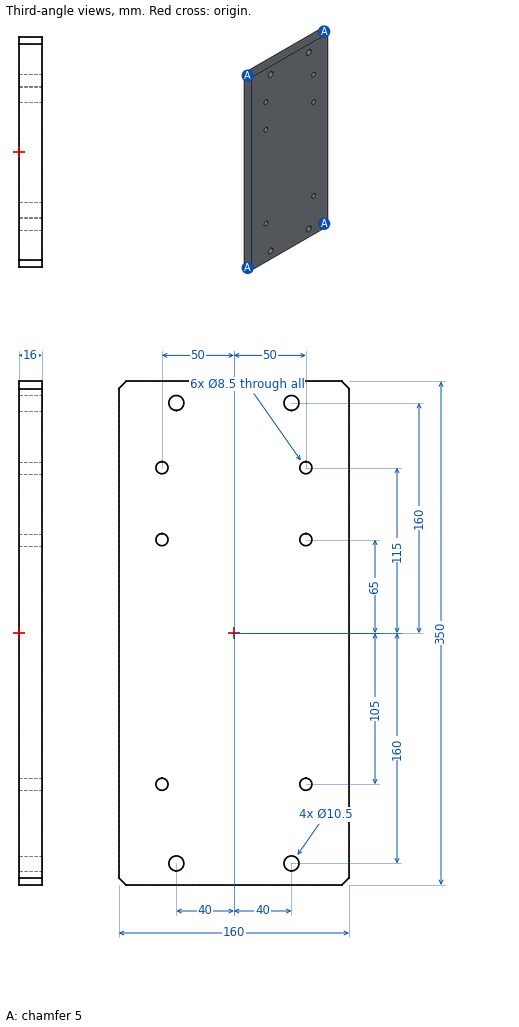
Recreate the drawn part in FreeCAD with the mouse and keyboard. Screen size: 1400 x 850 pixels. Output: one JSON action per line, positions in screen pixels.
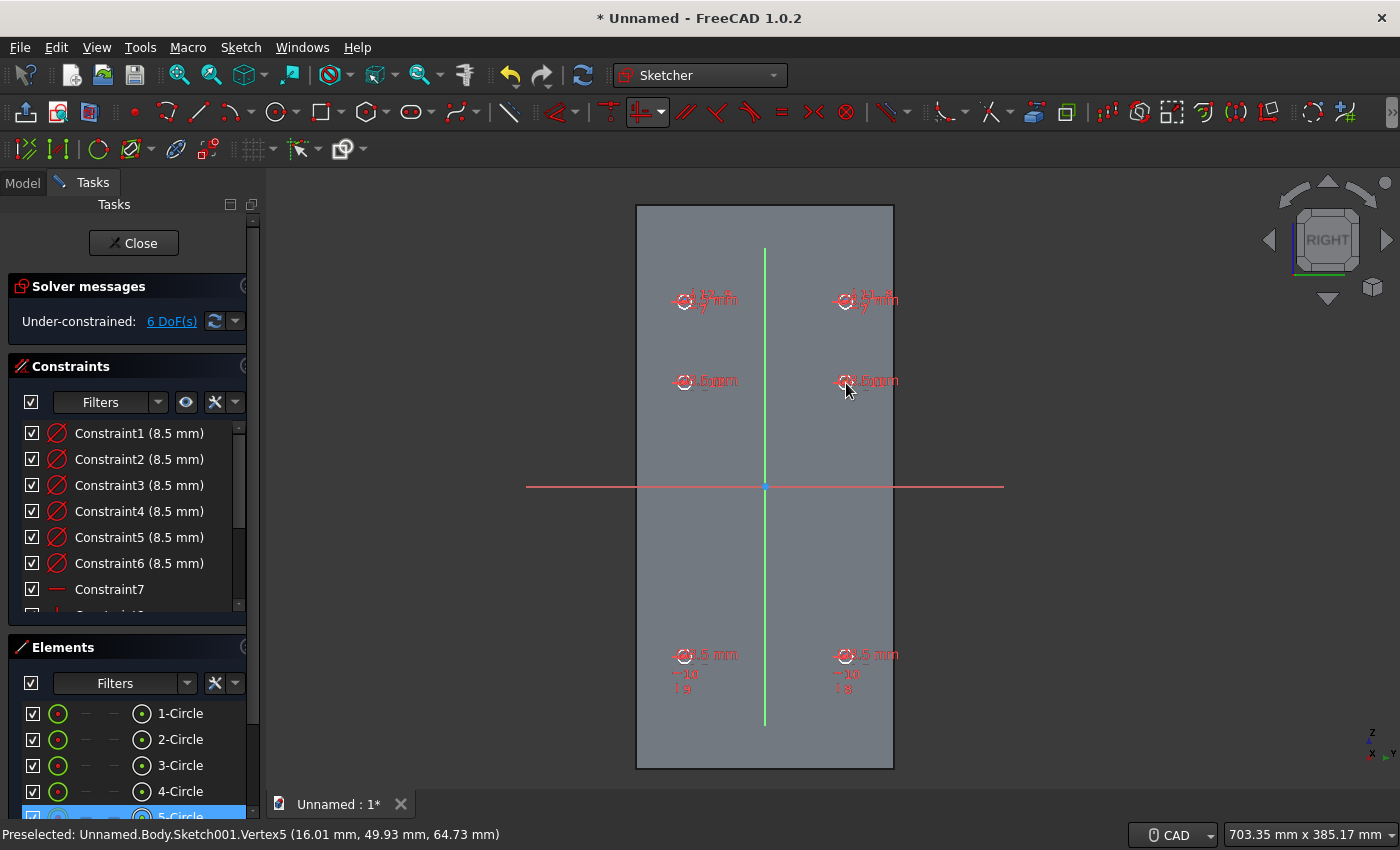
{"action": "left_click", "coordinate": [685, 383]}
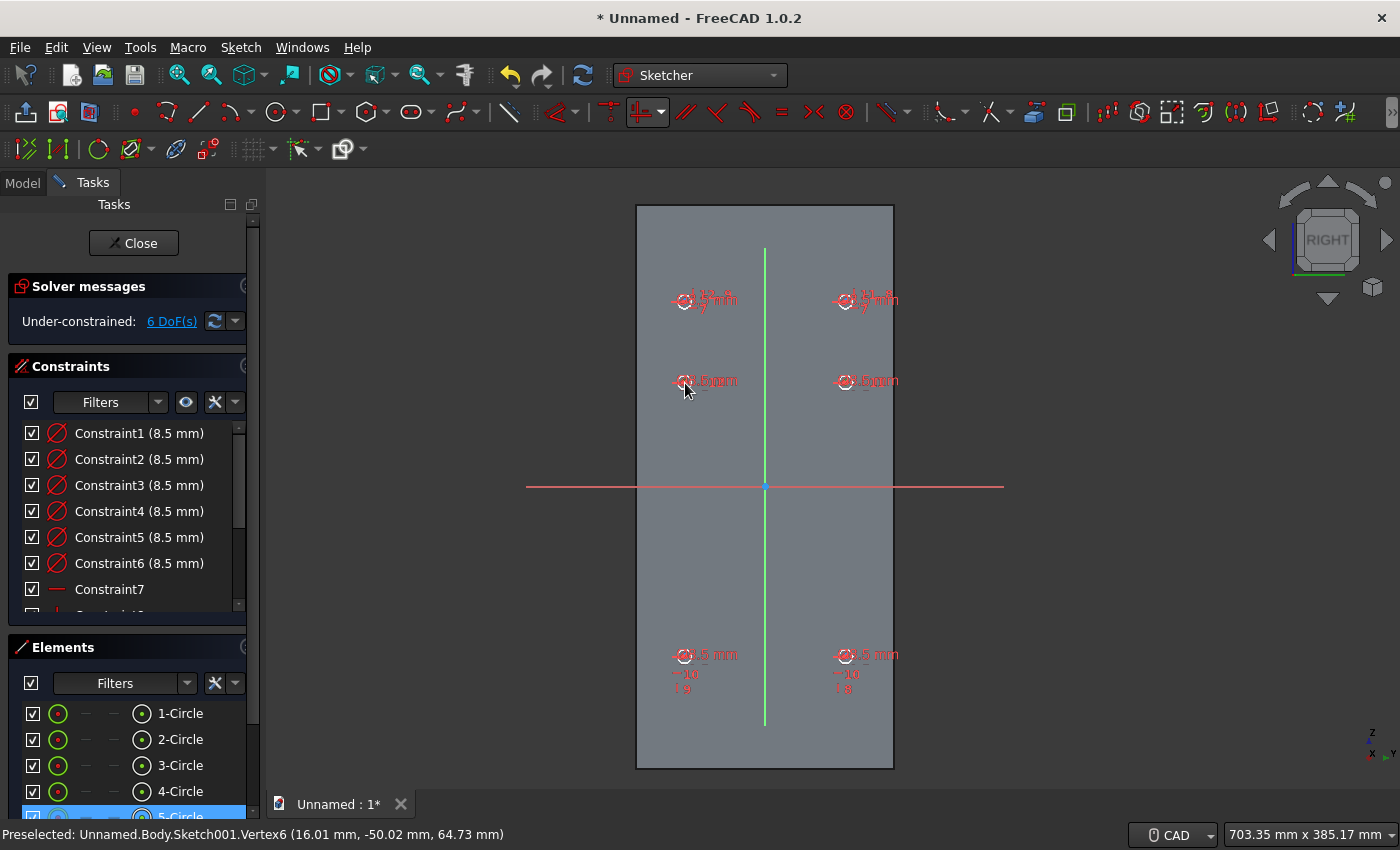
{"action": "key", "text": "h"}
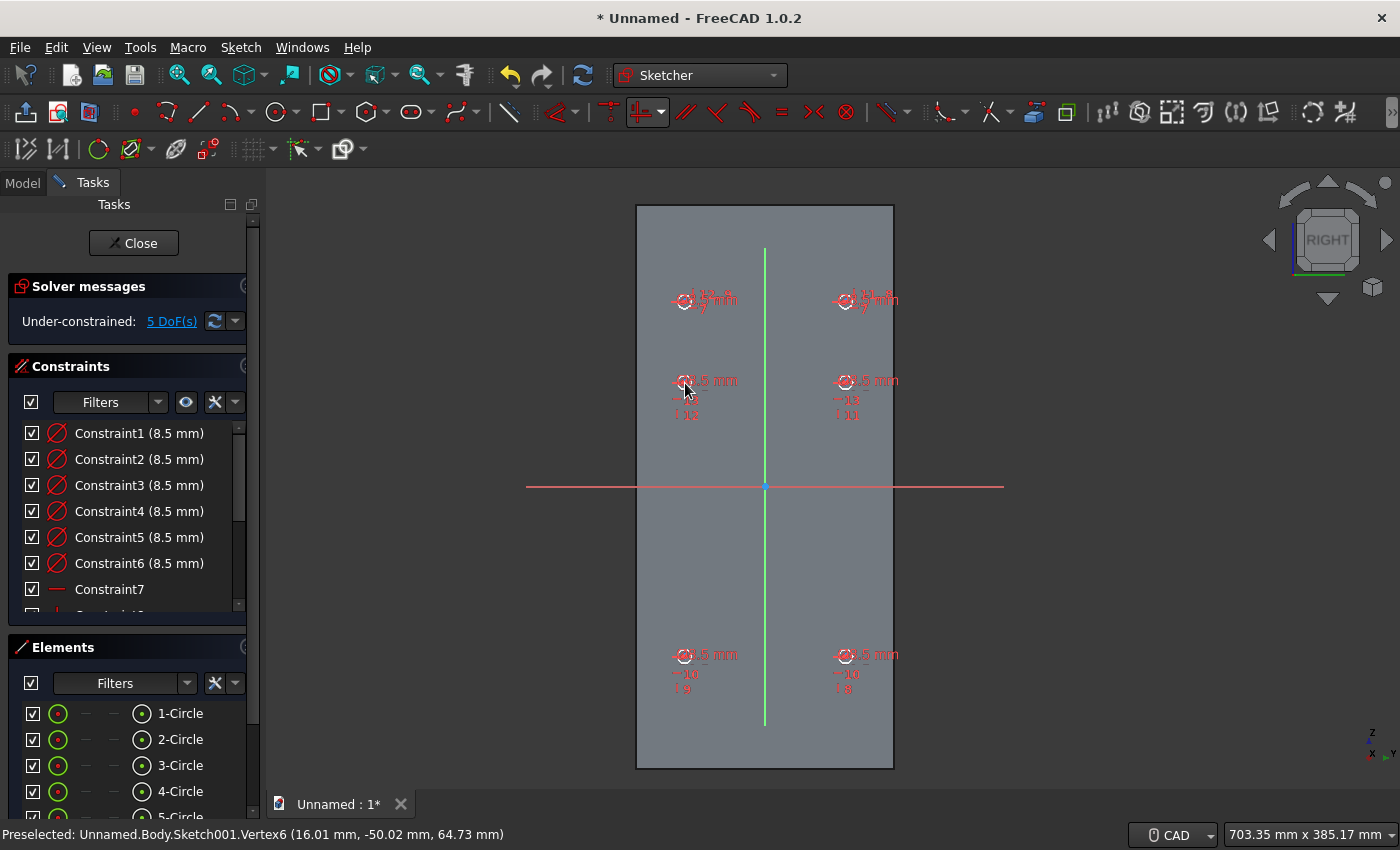
{"action": "left_click", "coordinate": [556, 112]}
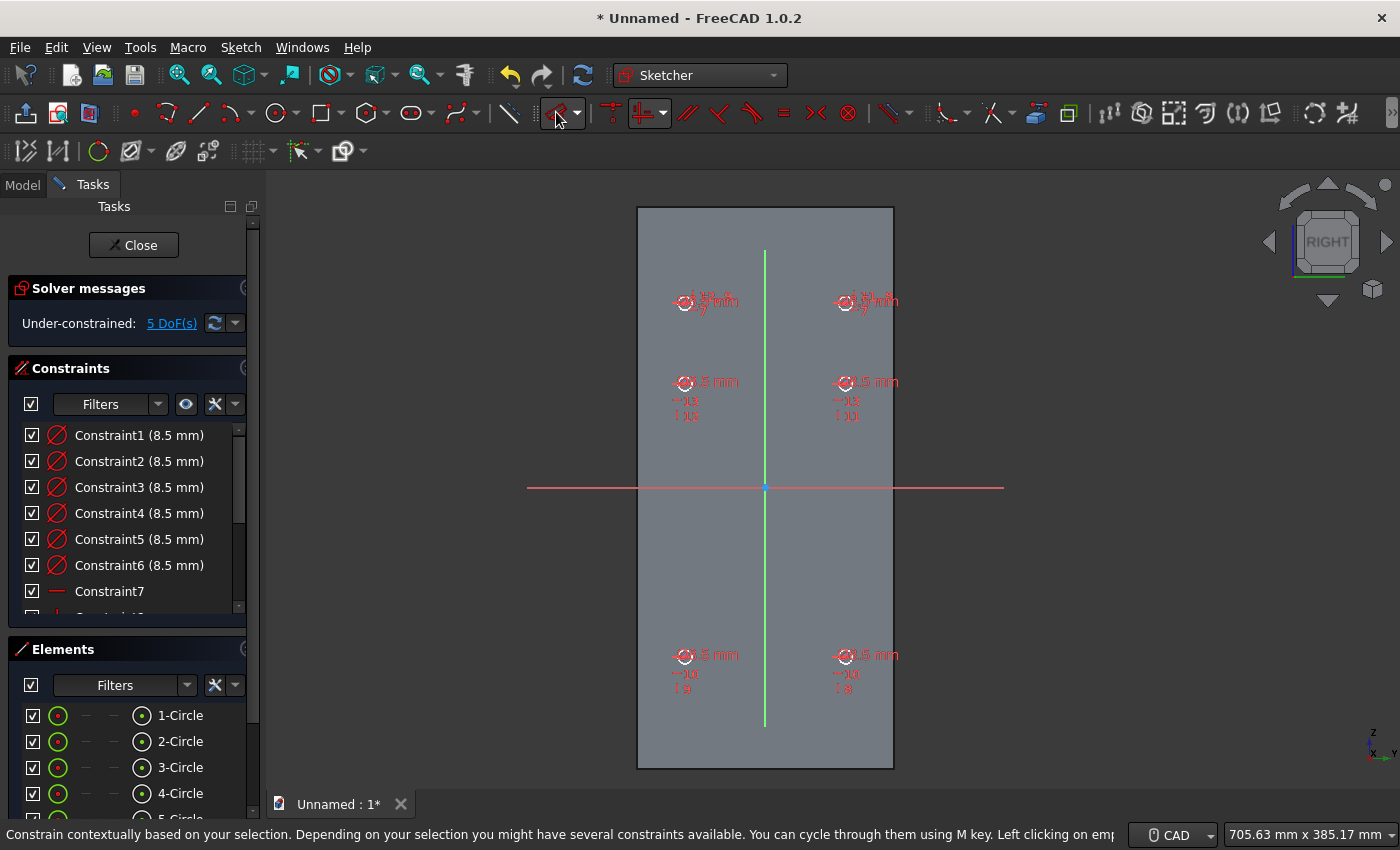
{"action": "left_click", "coordinate": [846, 303]}
{"action": "left_click", "coordinate": [805, 269]}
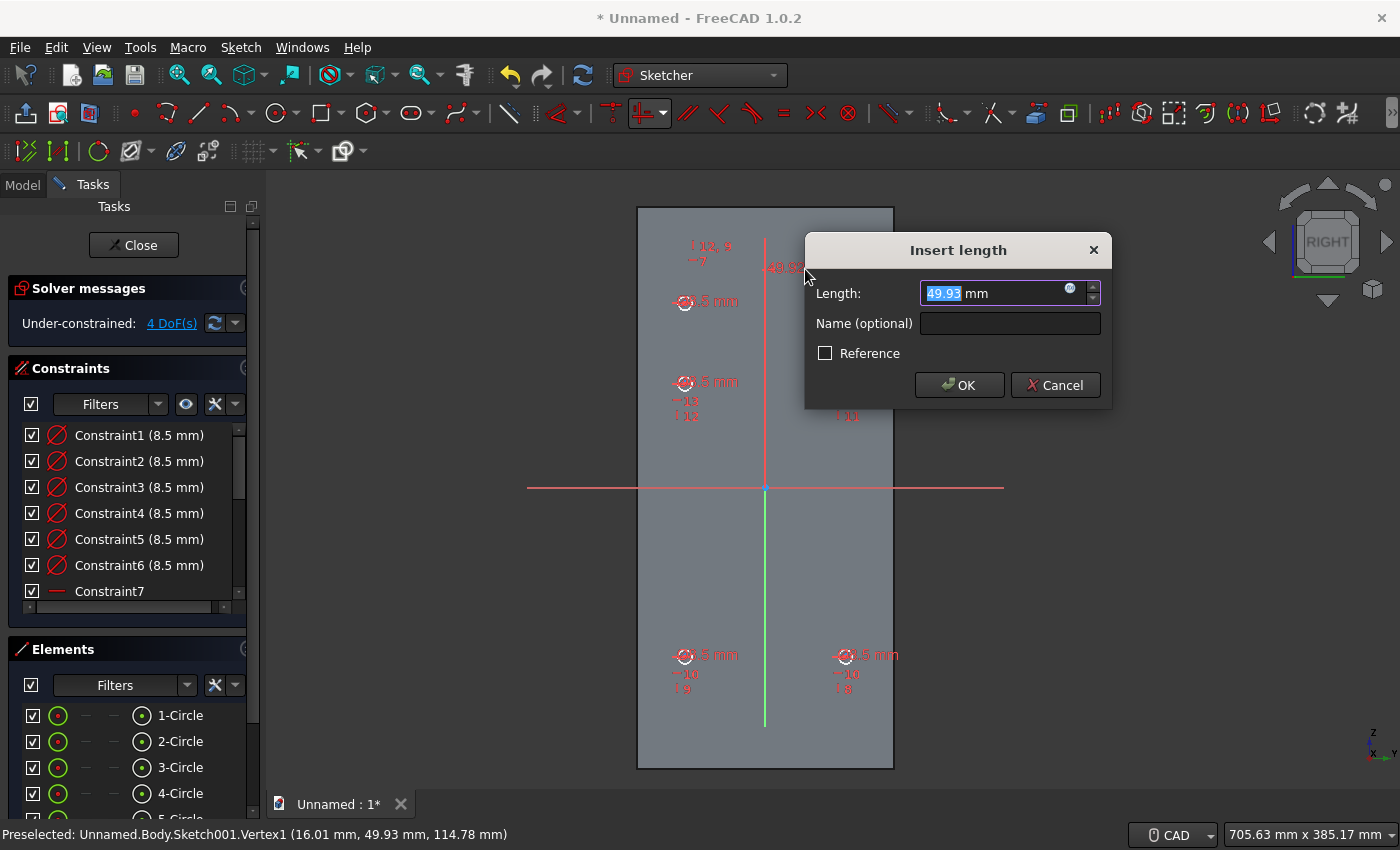
{"action": "type", "text": "50"}
{"action": "key", "text": "Return"}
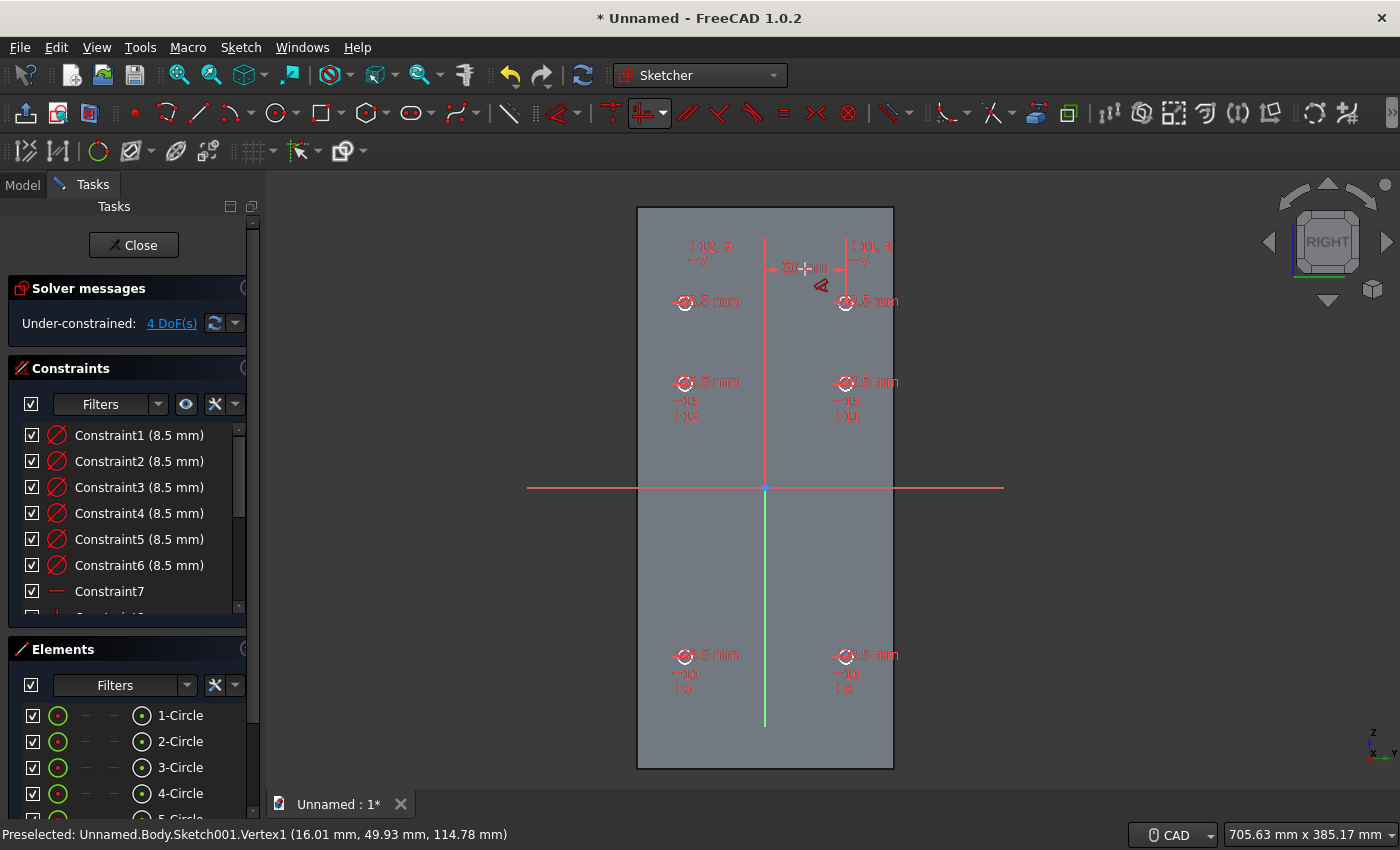
{"action": "left_click", "coordinate": [685, 303]}
{"action": "left_click", "coordinate": [725, 269]}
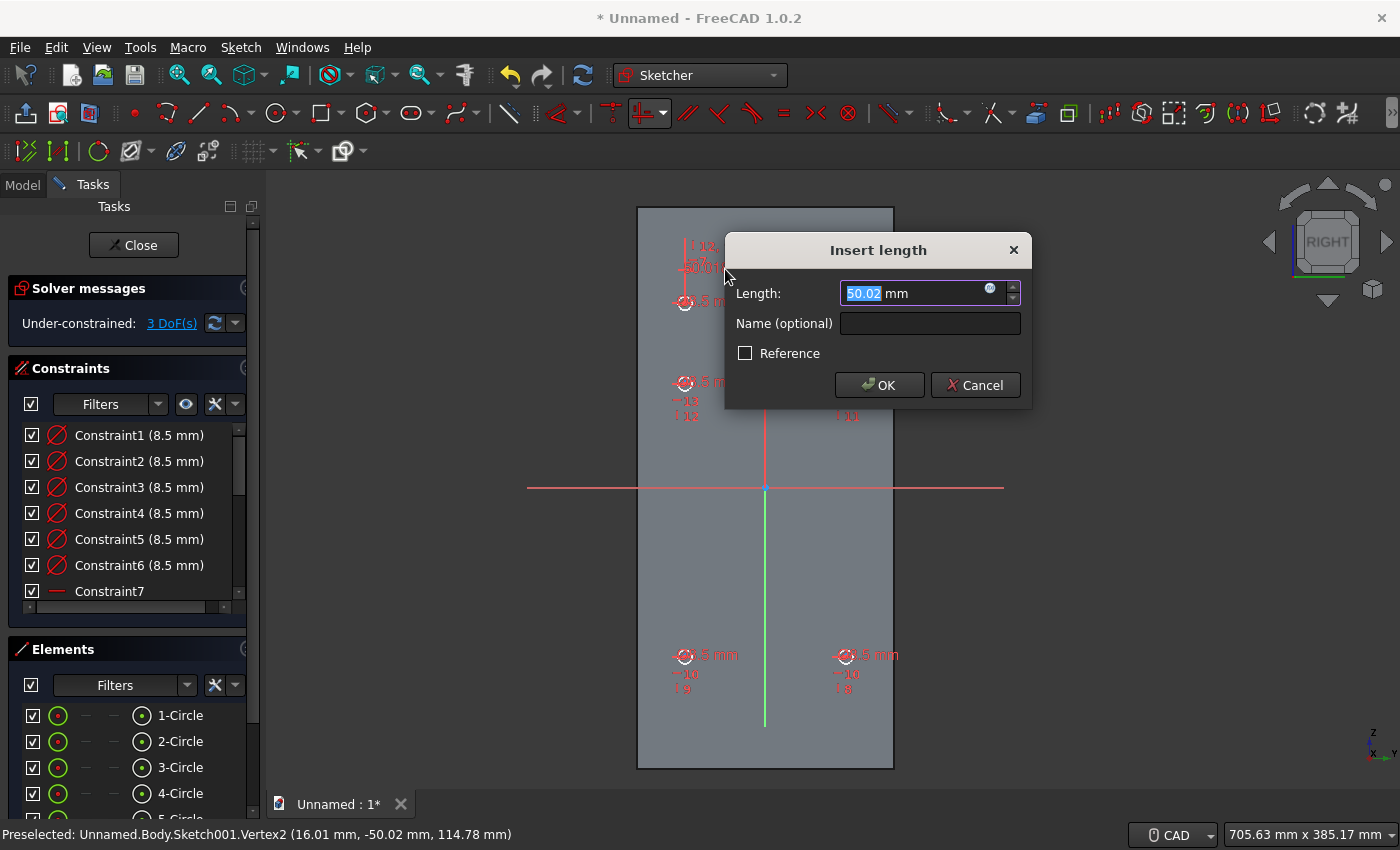
{"action": "type", "text": "50"}
{"action": "key", "text": "Return"}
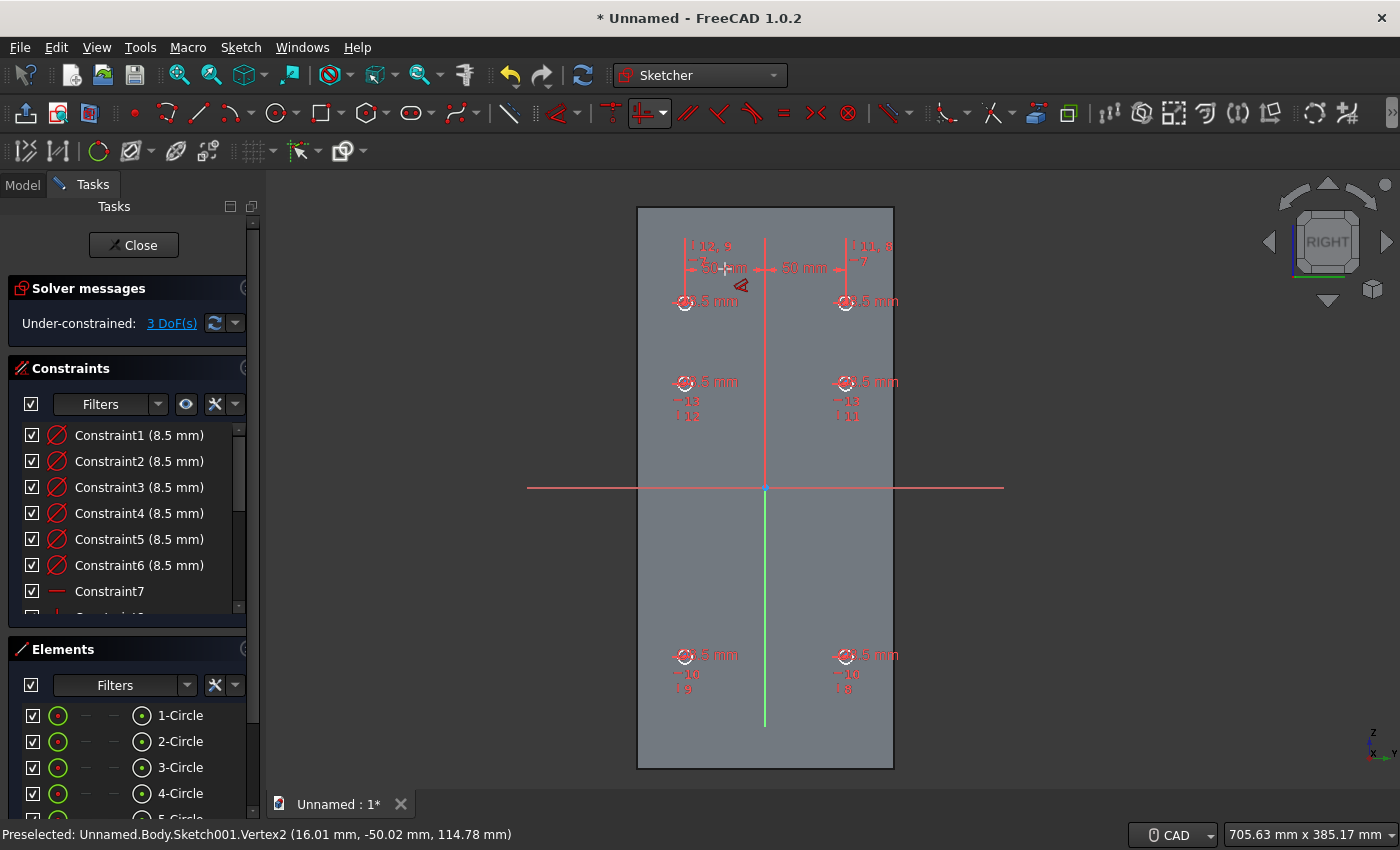
{"action": "left_click", "coordinate": [846, 384]}
{"action": "left_click", "coordinate": [880, 436]}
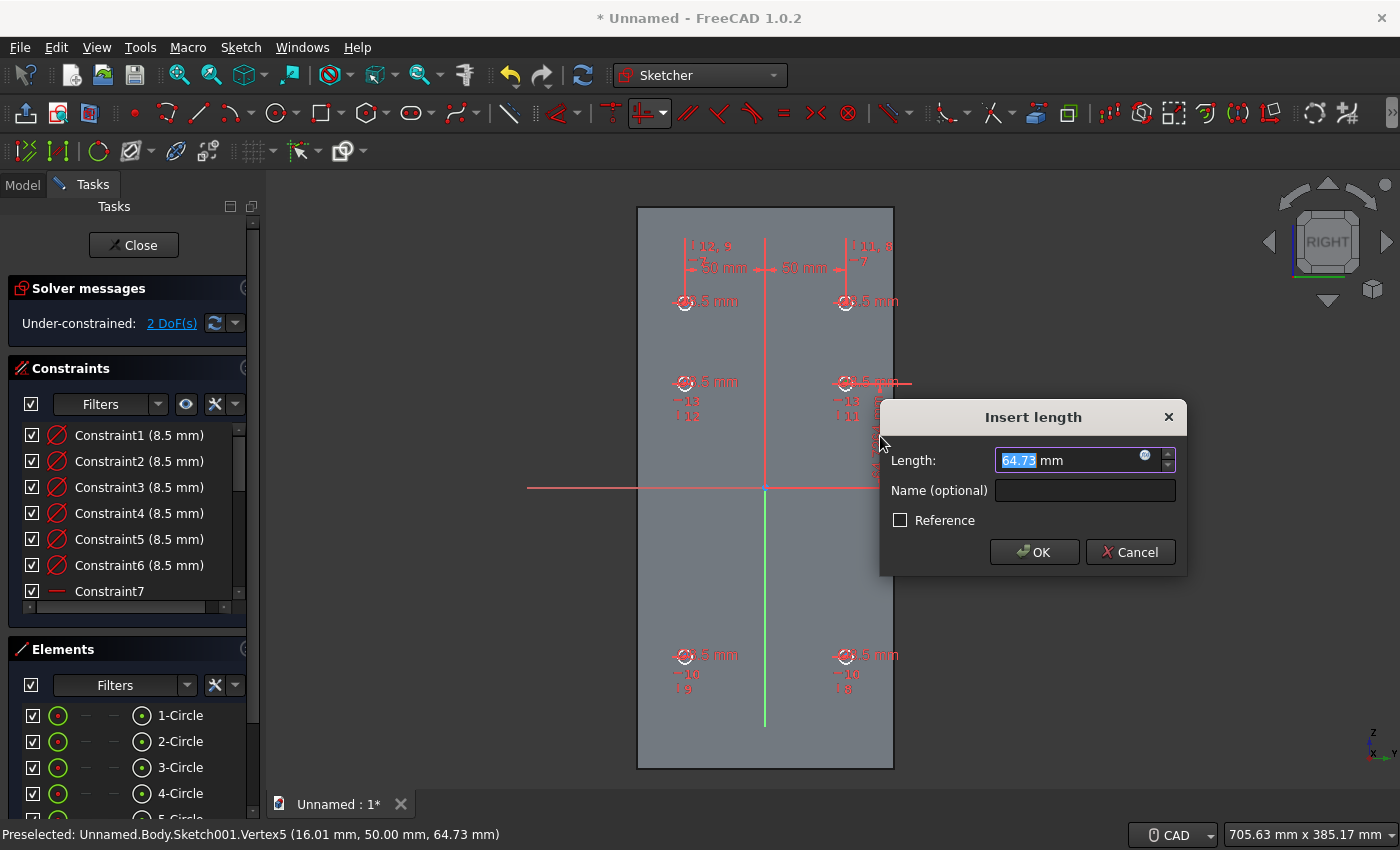
{"action": "type", "text": "65"}
{"action": "key", "text": "Return"}